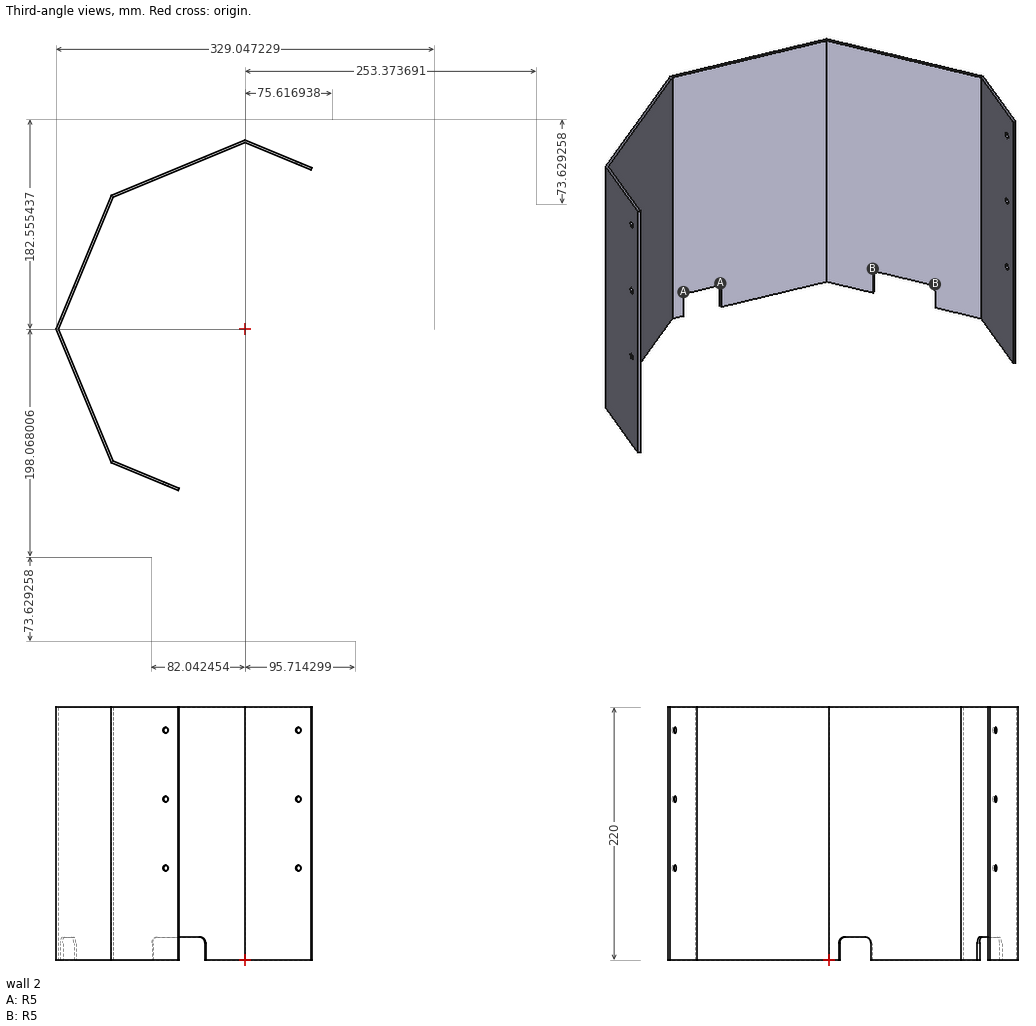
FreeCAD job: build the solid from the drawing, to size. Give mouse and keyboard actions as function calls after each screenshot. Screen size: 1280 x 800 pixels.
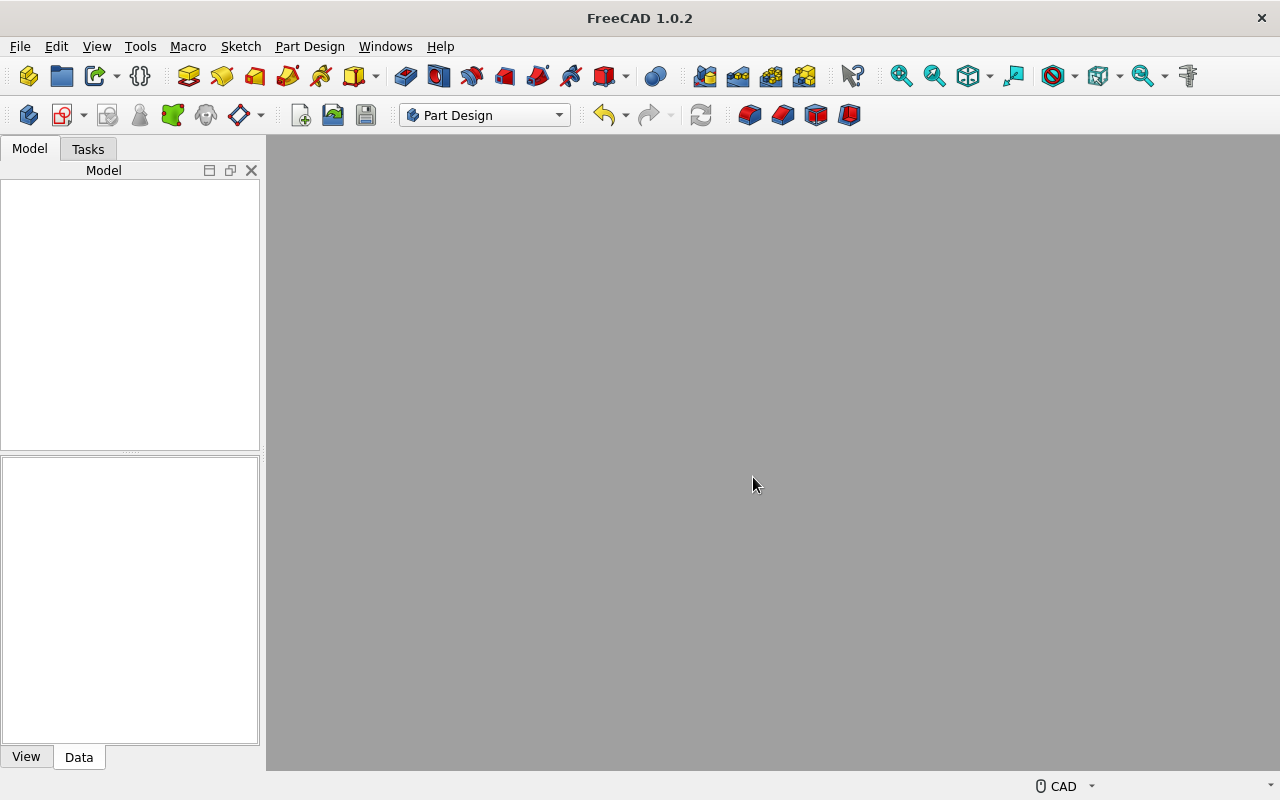
click(300, 116)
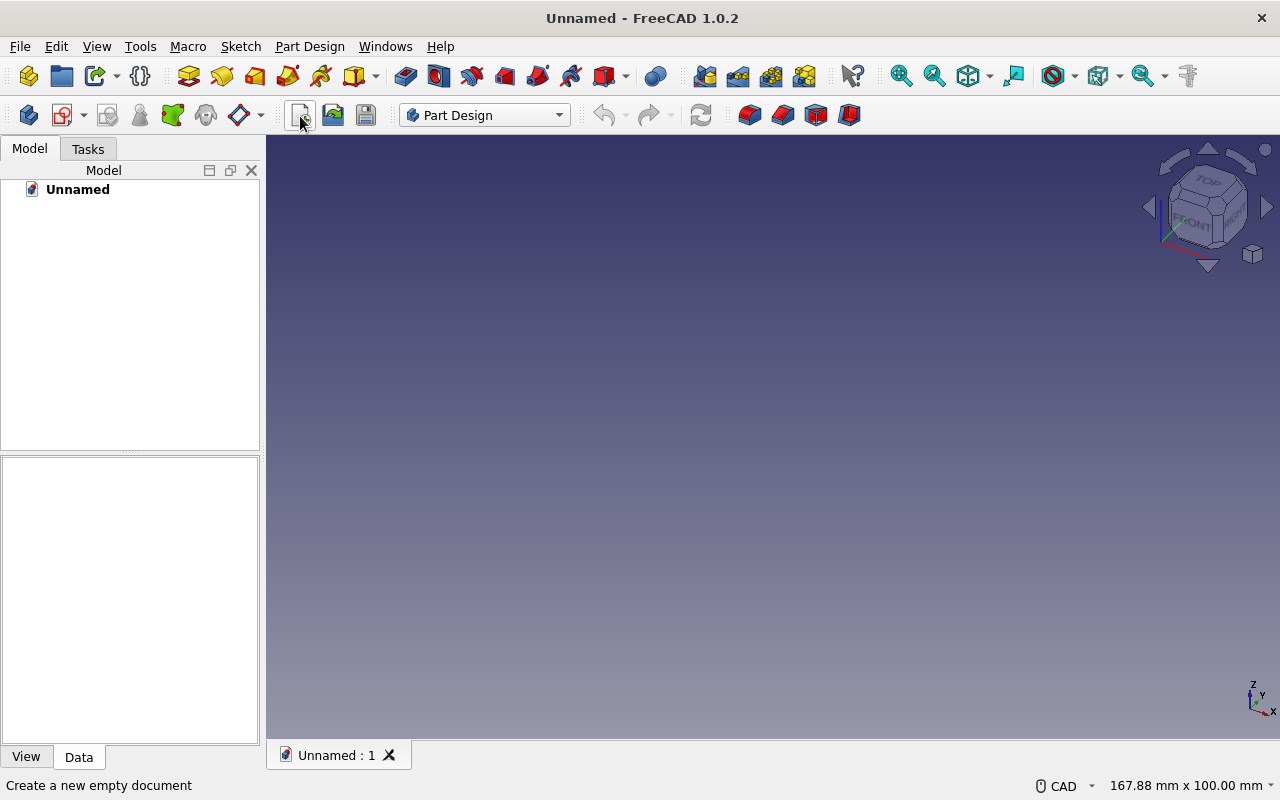
click(62, 116)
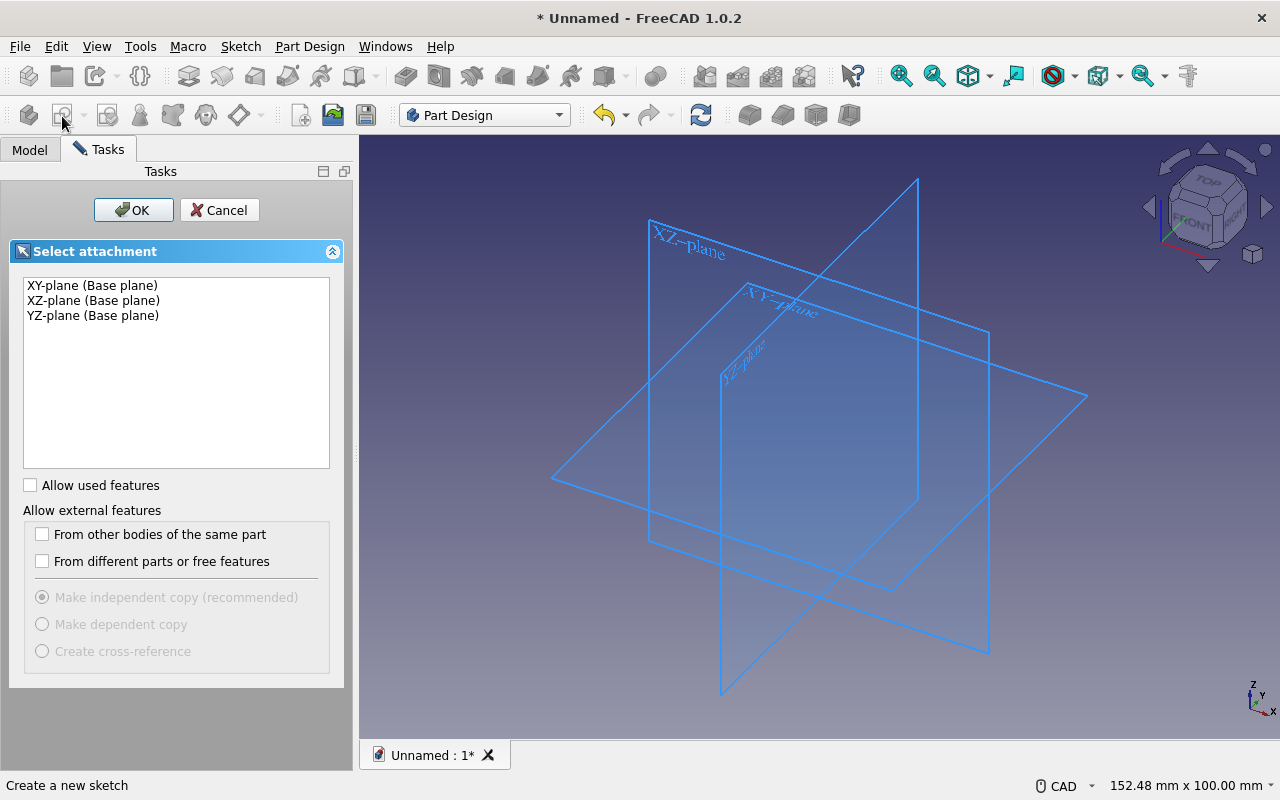
click(84, 286)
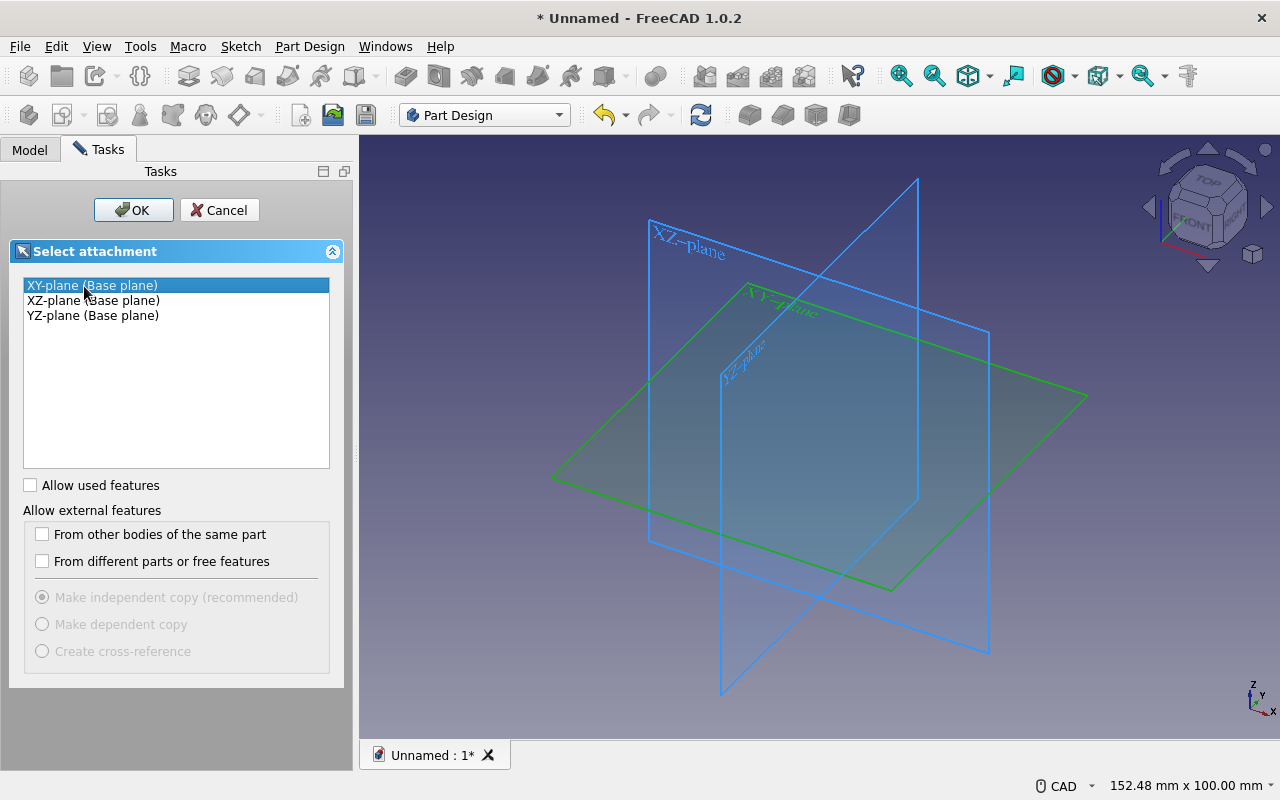
click(134, 210)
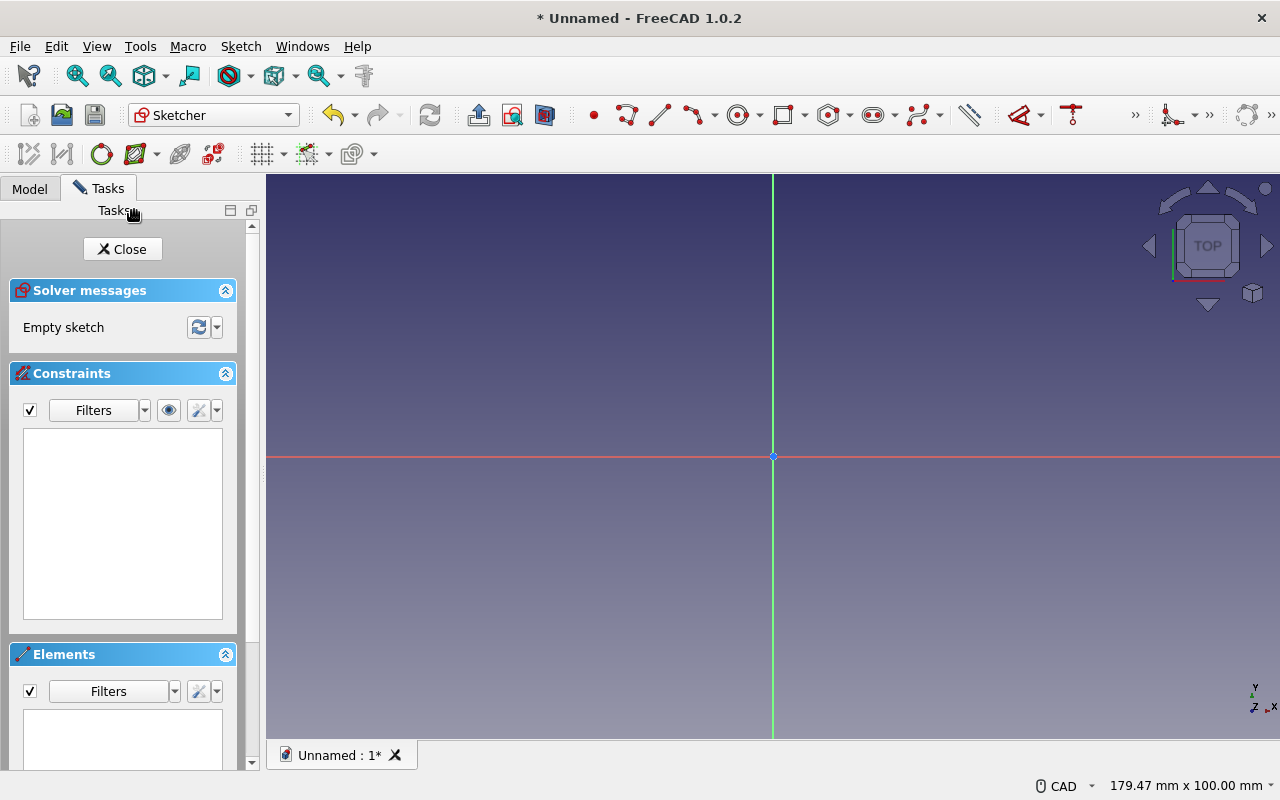
scroll(687, 456, down, 8)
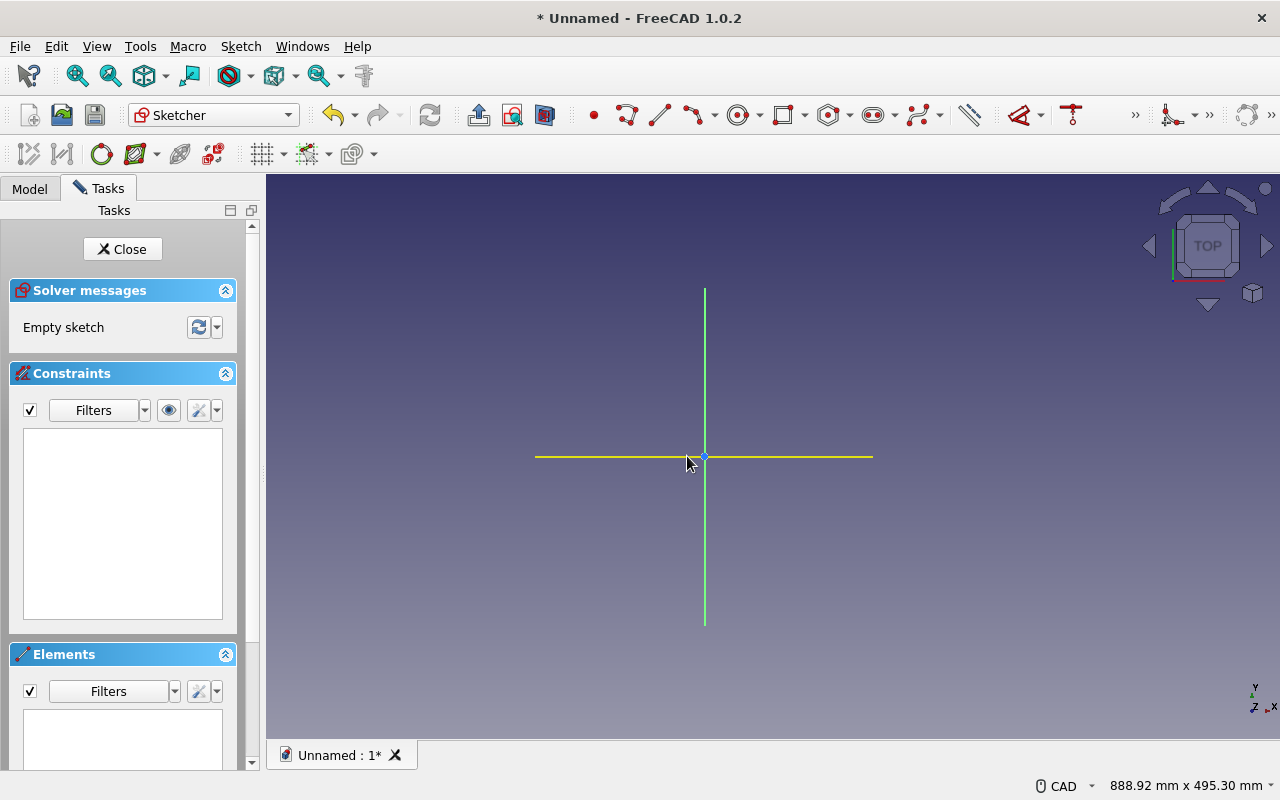
click(850, 116)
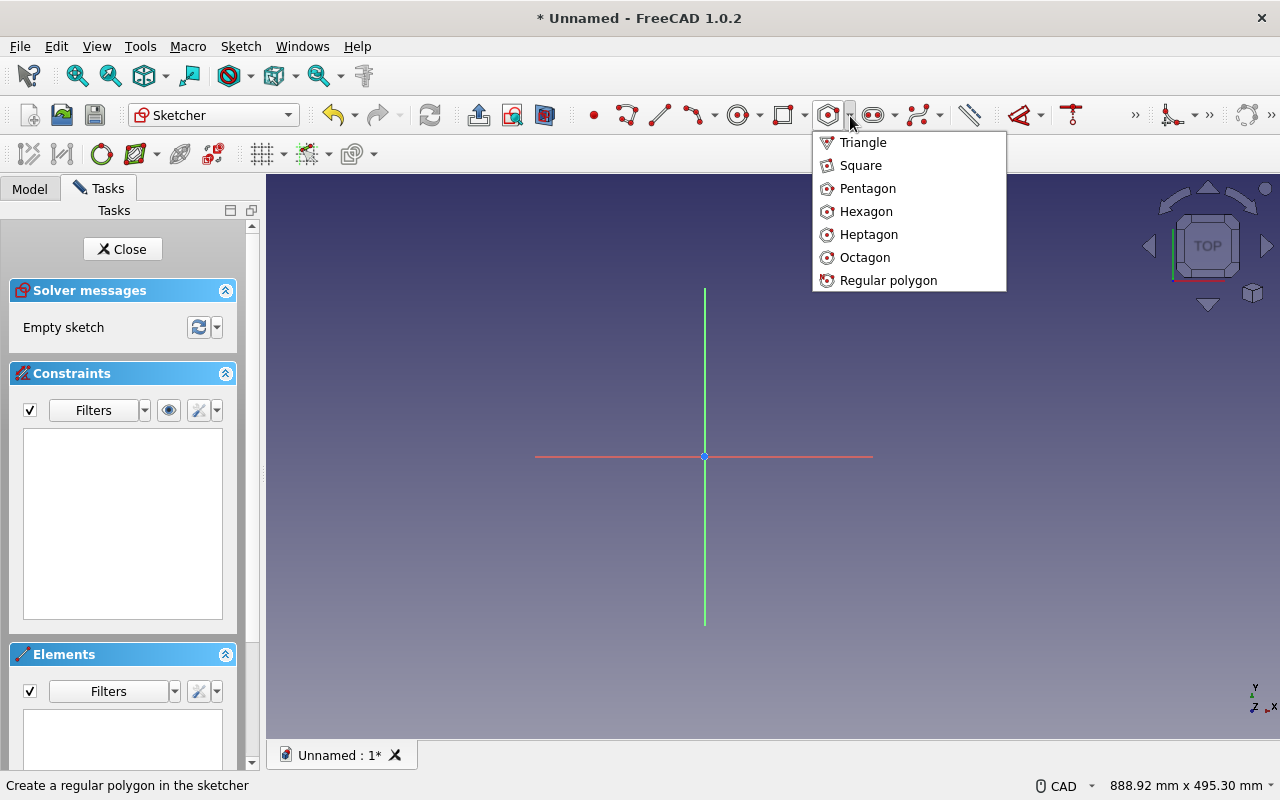
click(910, 258)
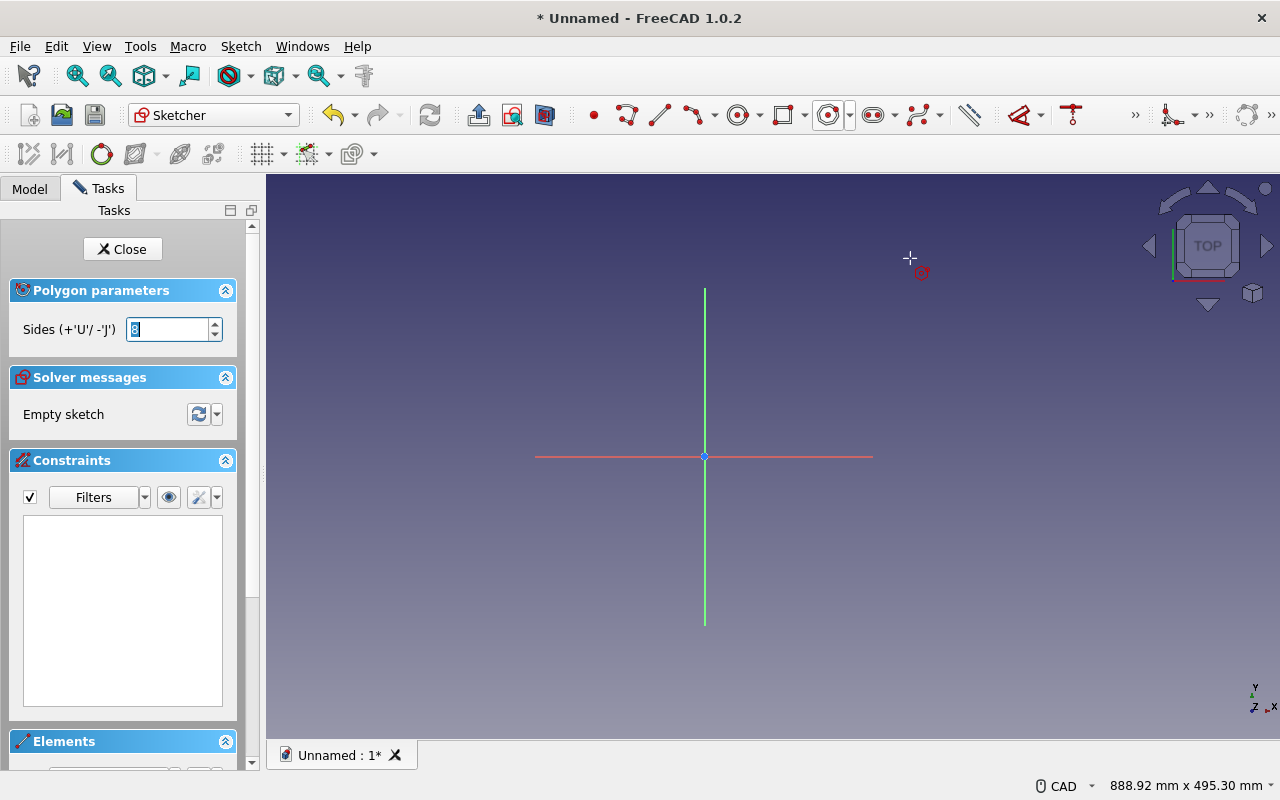
click(705, 456)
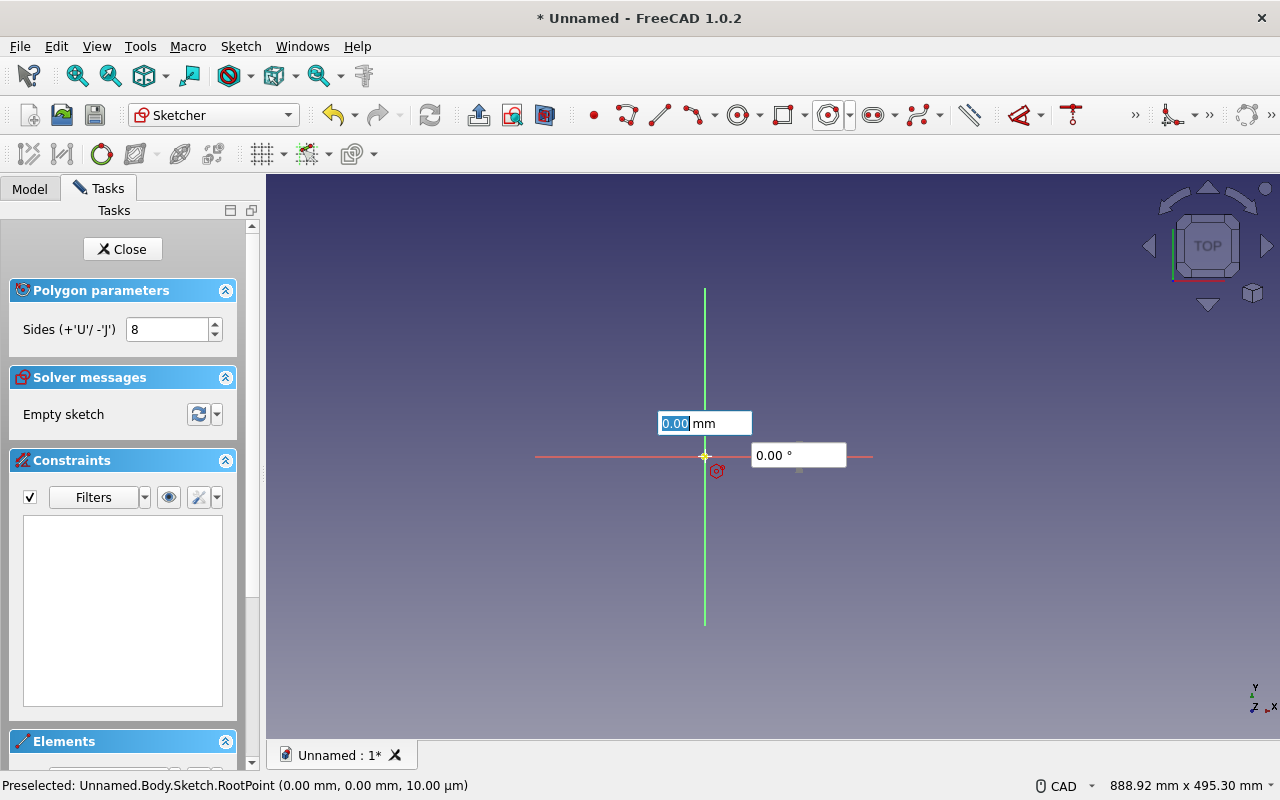
click(517, 456)
right_click(517, 456)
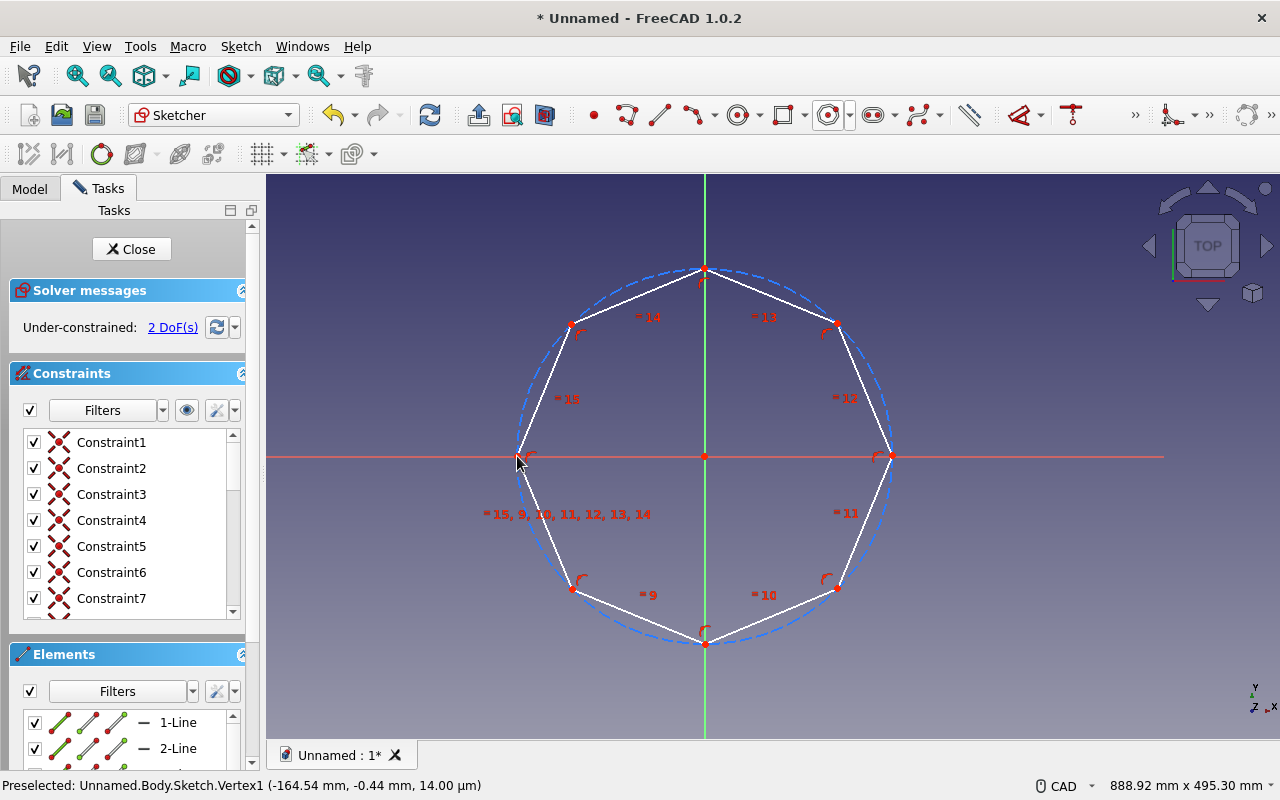
click(517, 457)